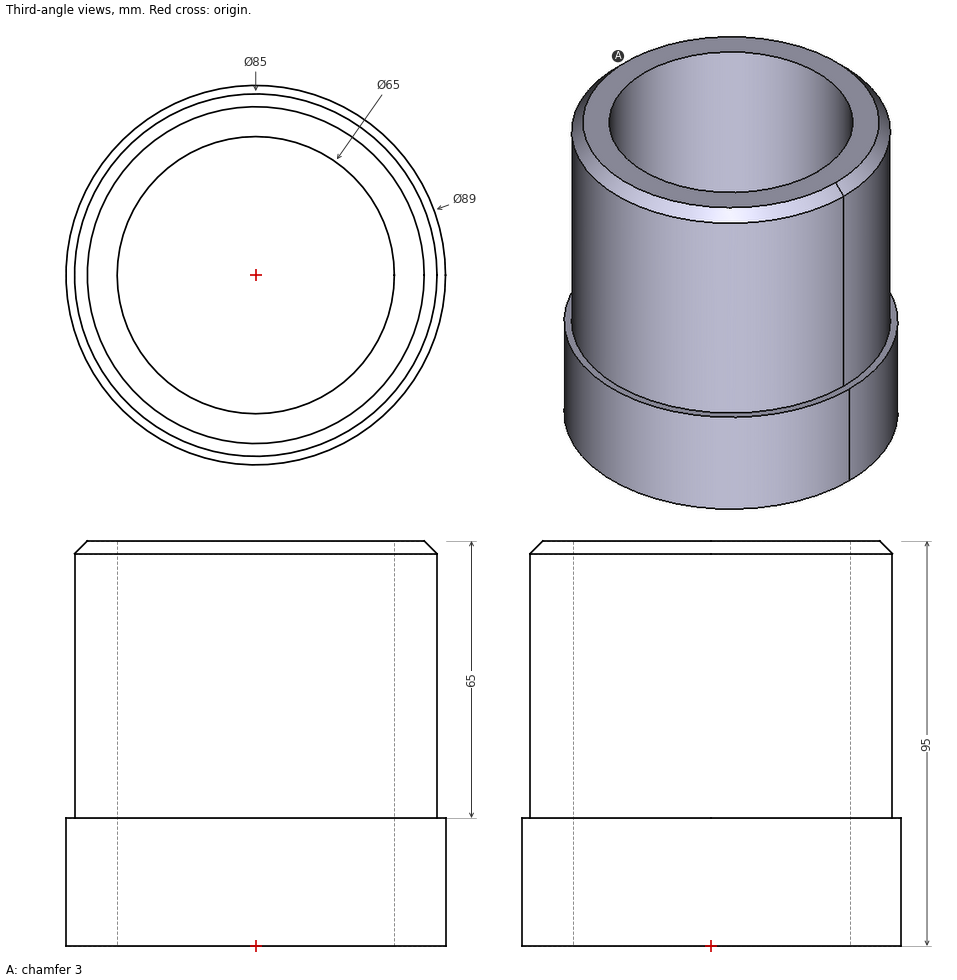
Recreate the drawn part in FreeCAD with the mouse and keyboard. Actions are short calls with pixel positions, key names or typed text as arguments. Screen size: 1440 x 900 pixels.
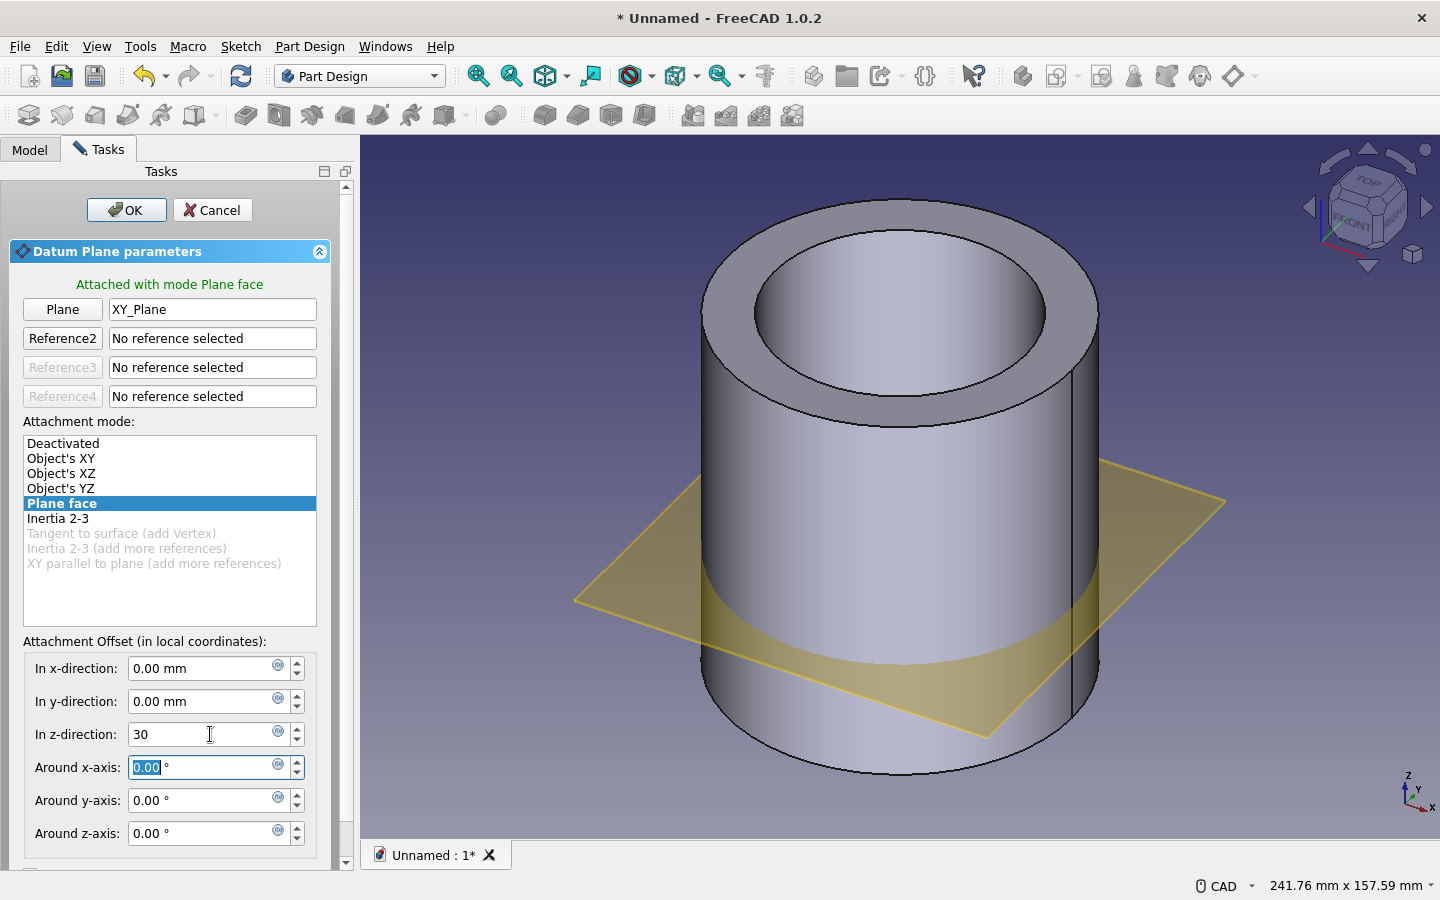
click(127, 210)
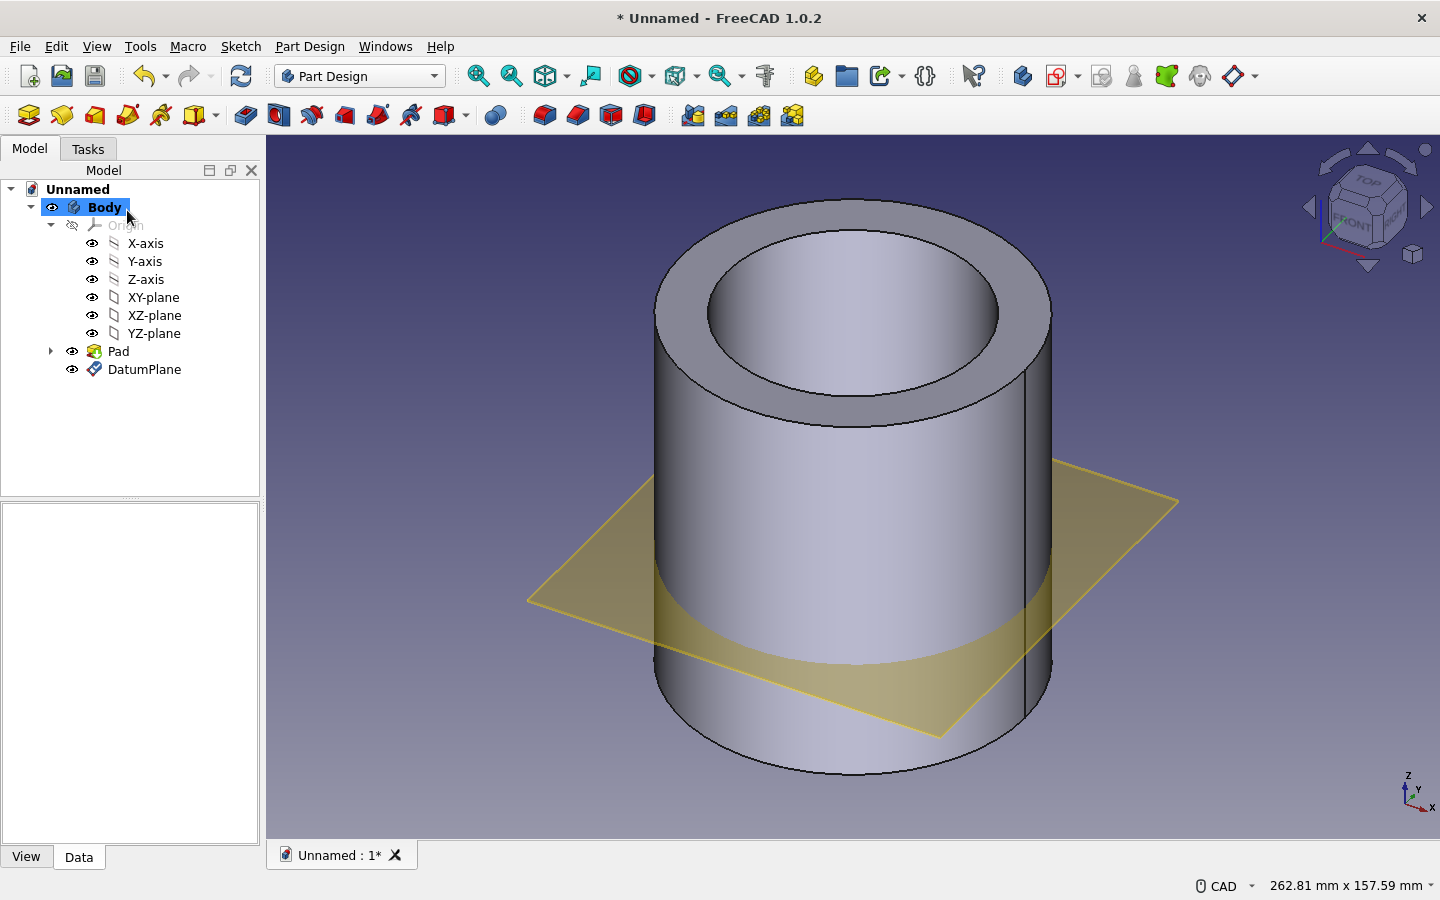
click(117, 369)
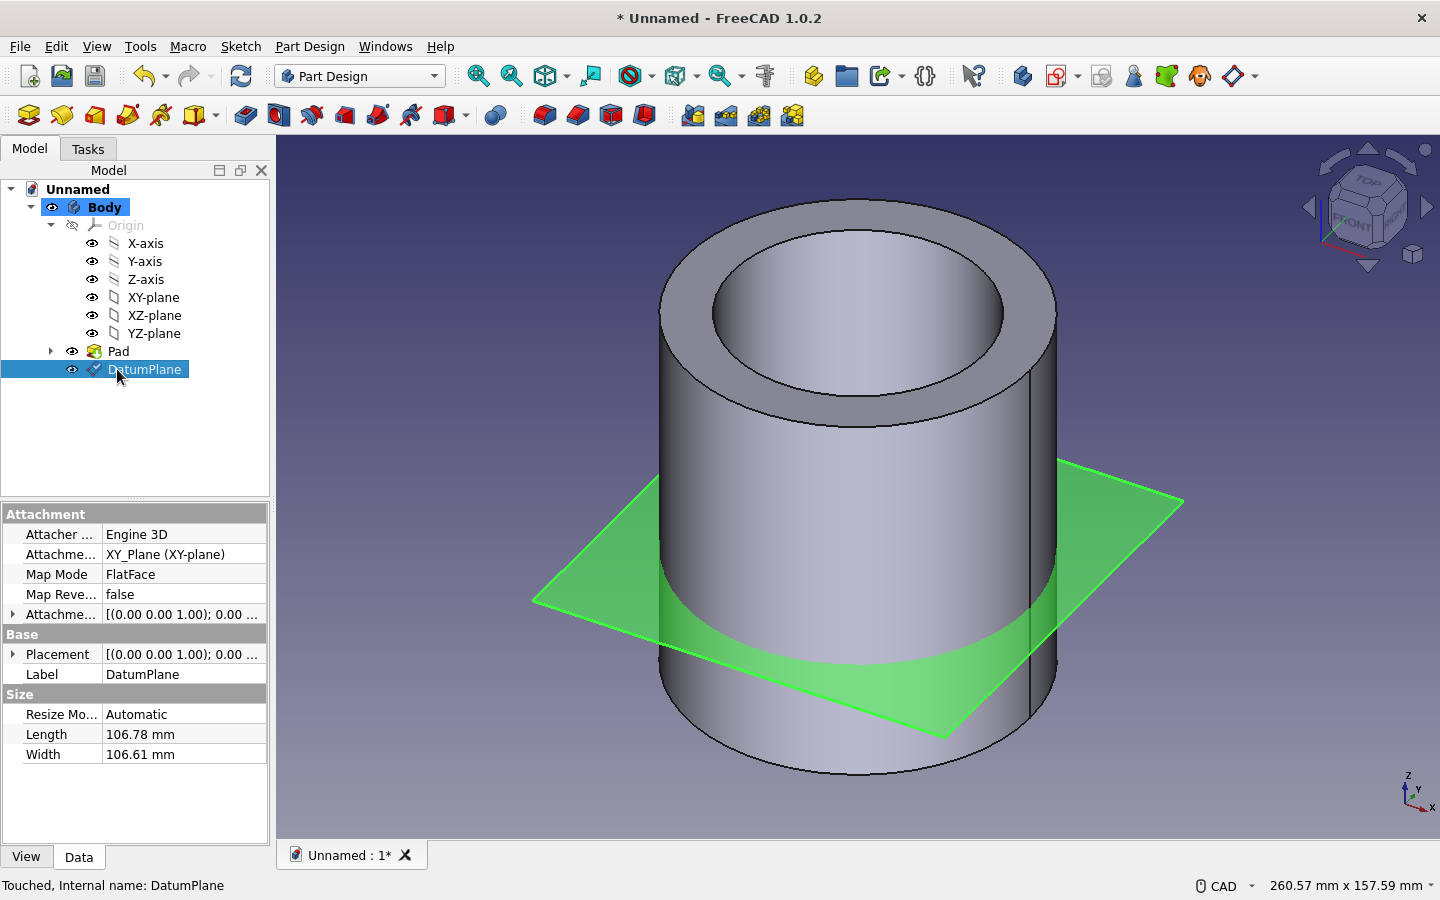
click(1056, 76)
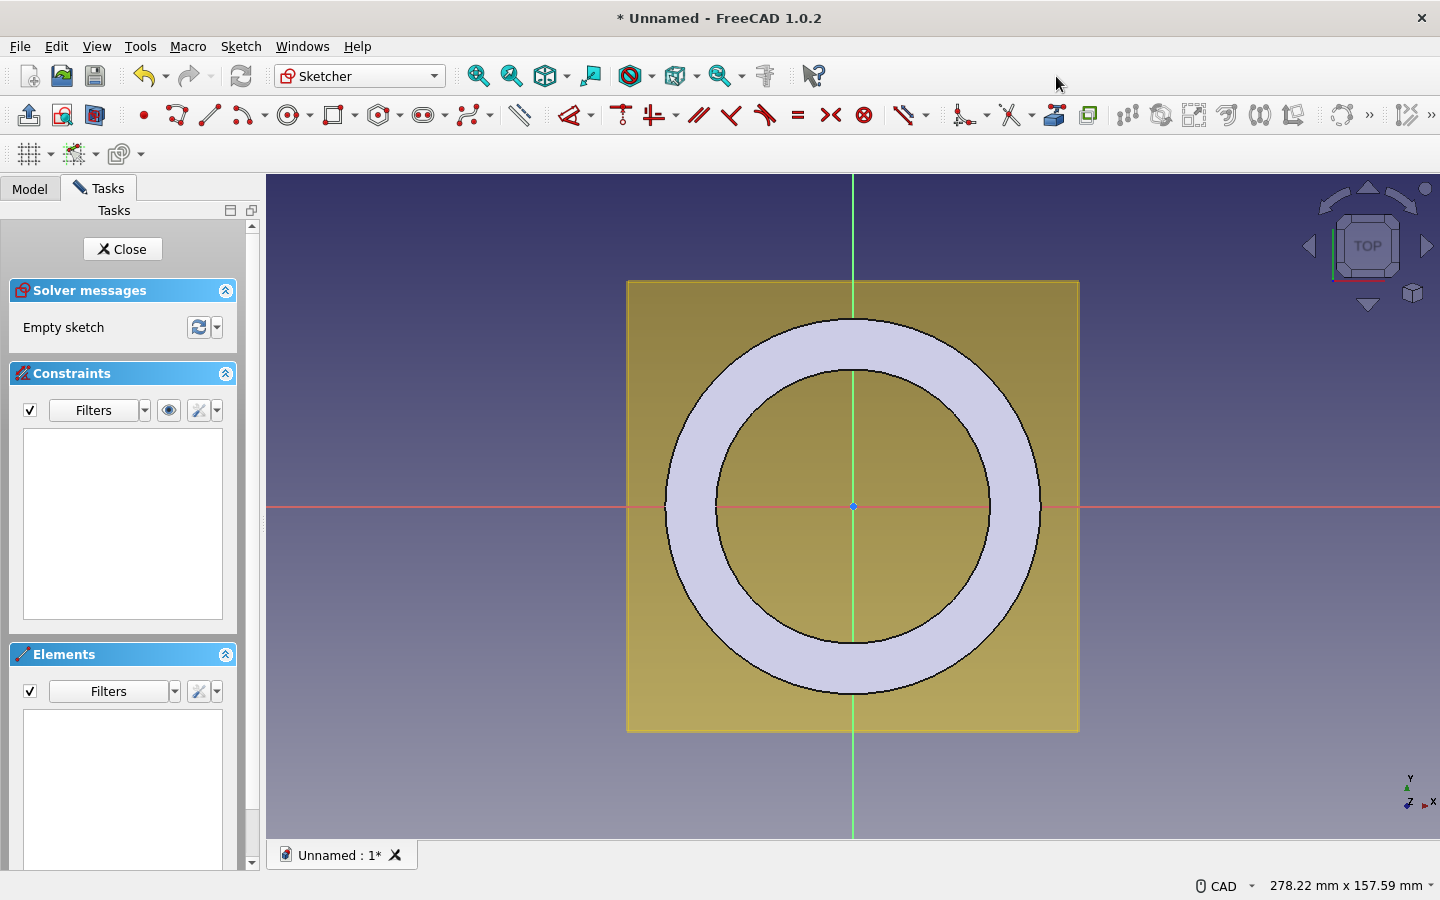
click(95, 116)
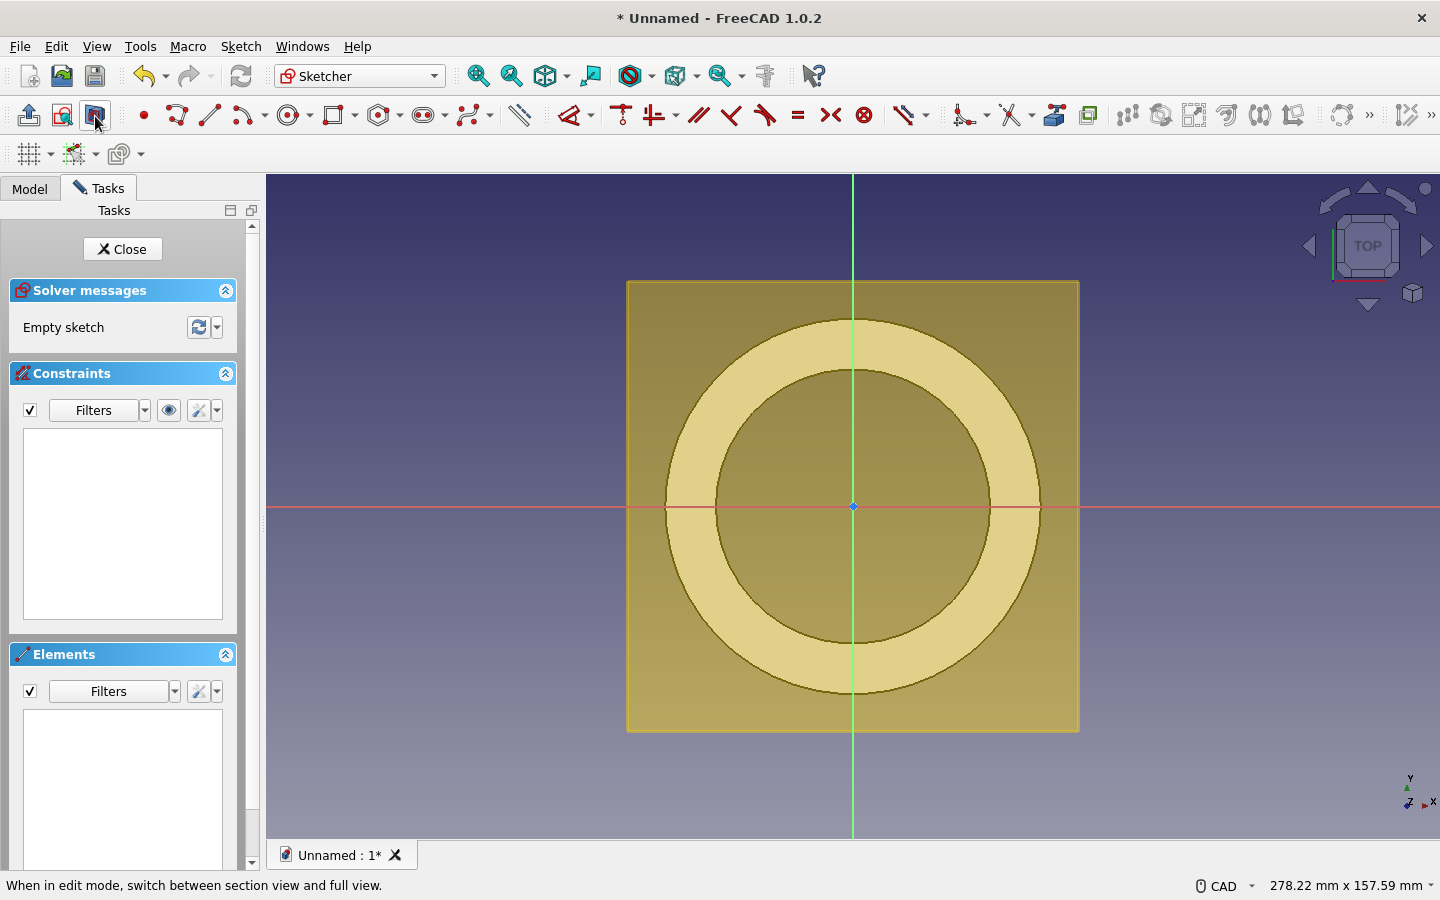
click(288, 116)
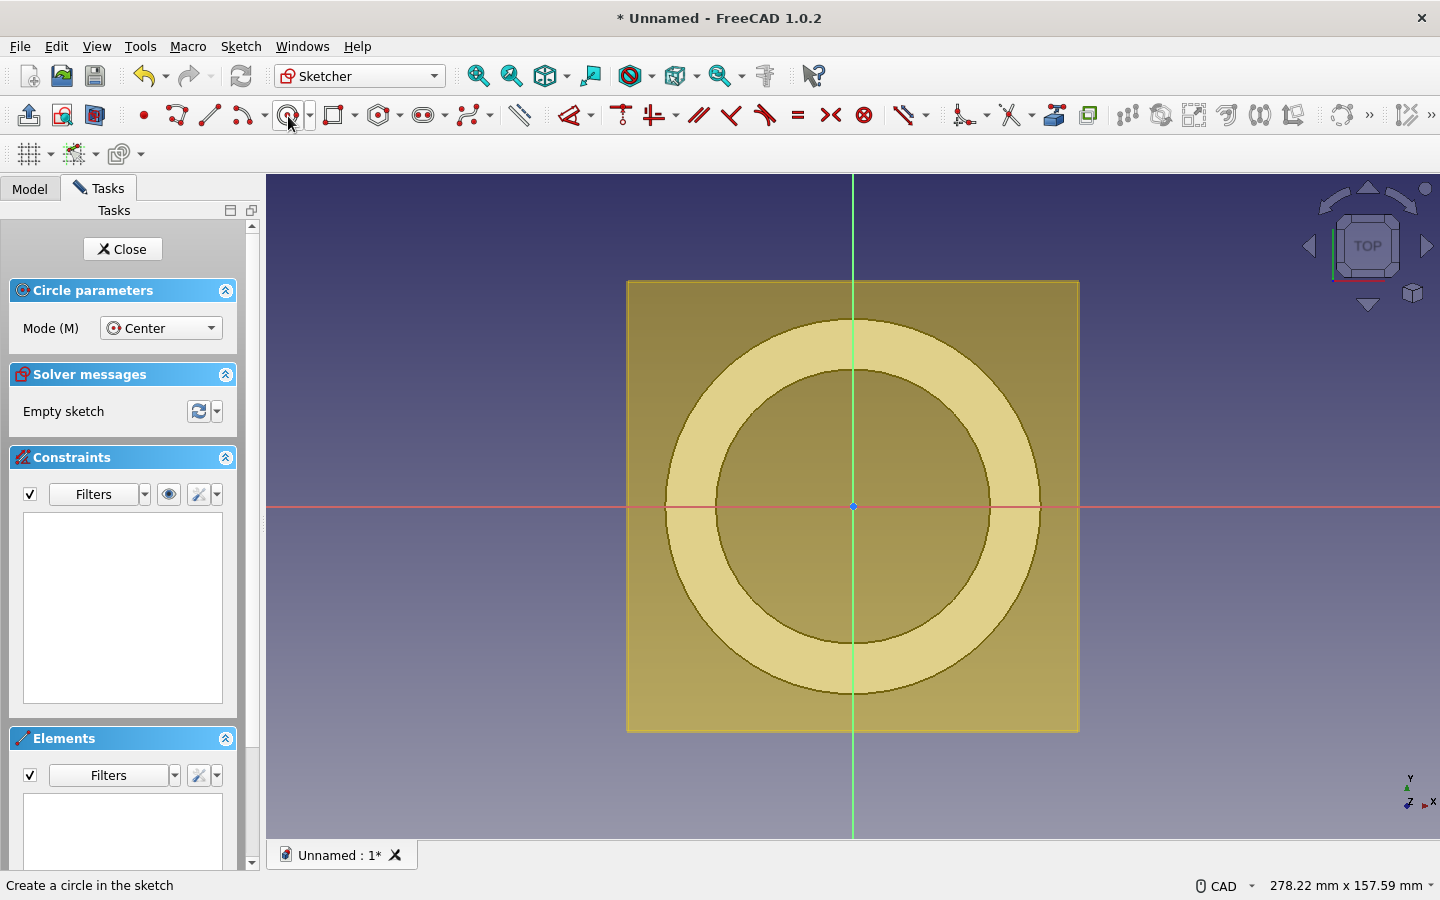
click(853, 506)
click(986, 374)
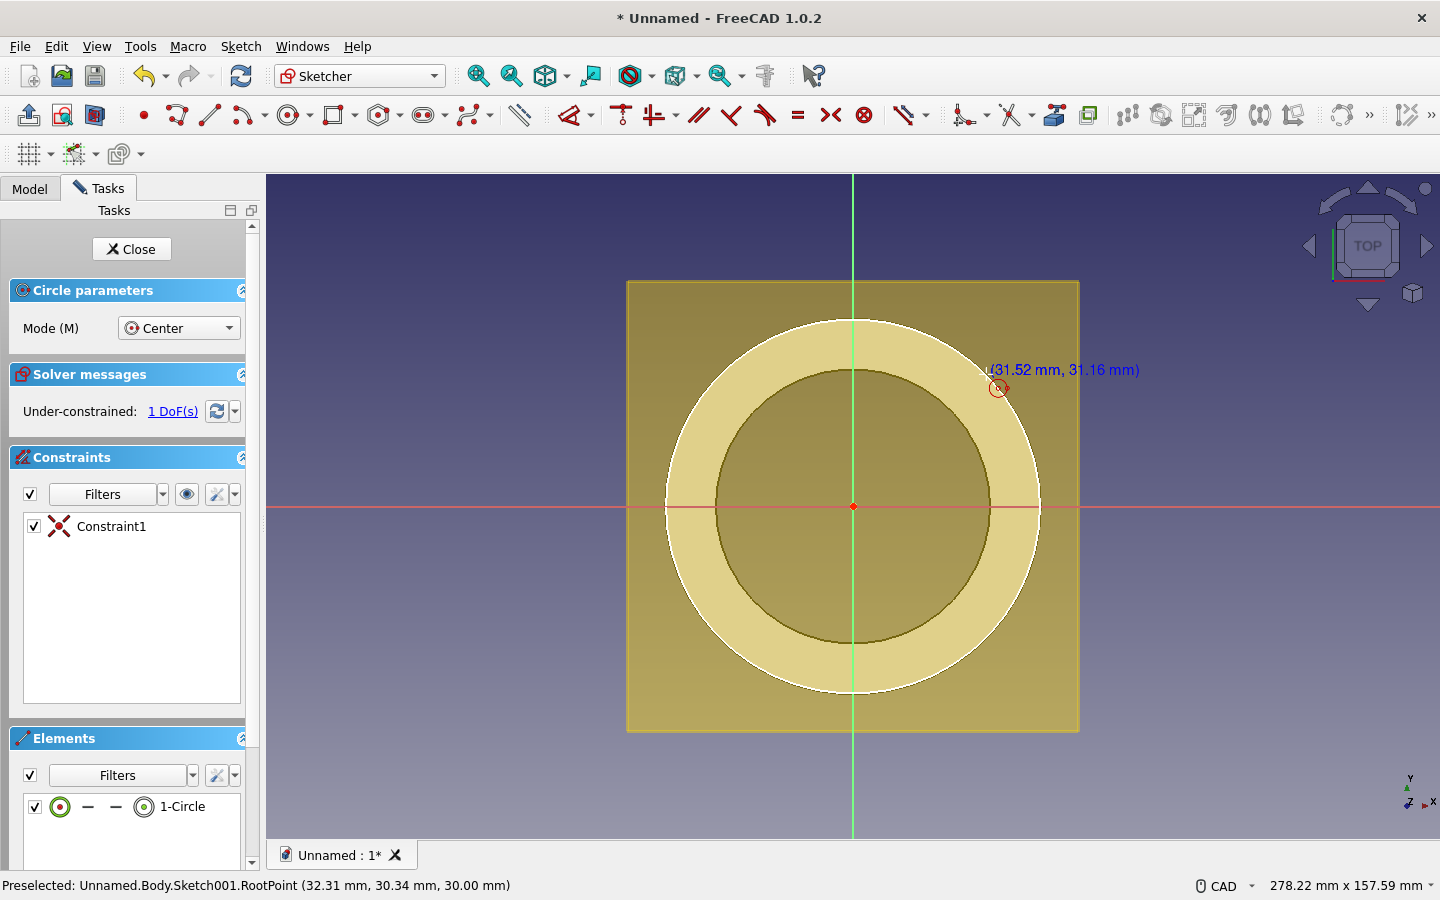
click(853, 506)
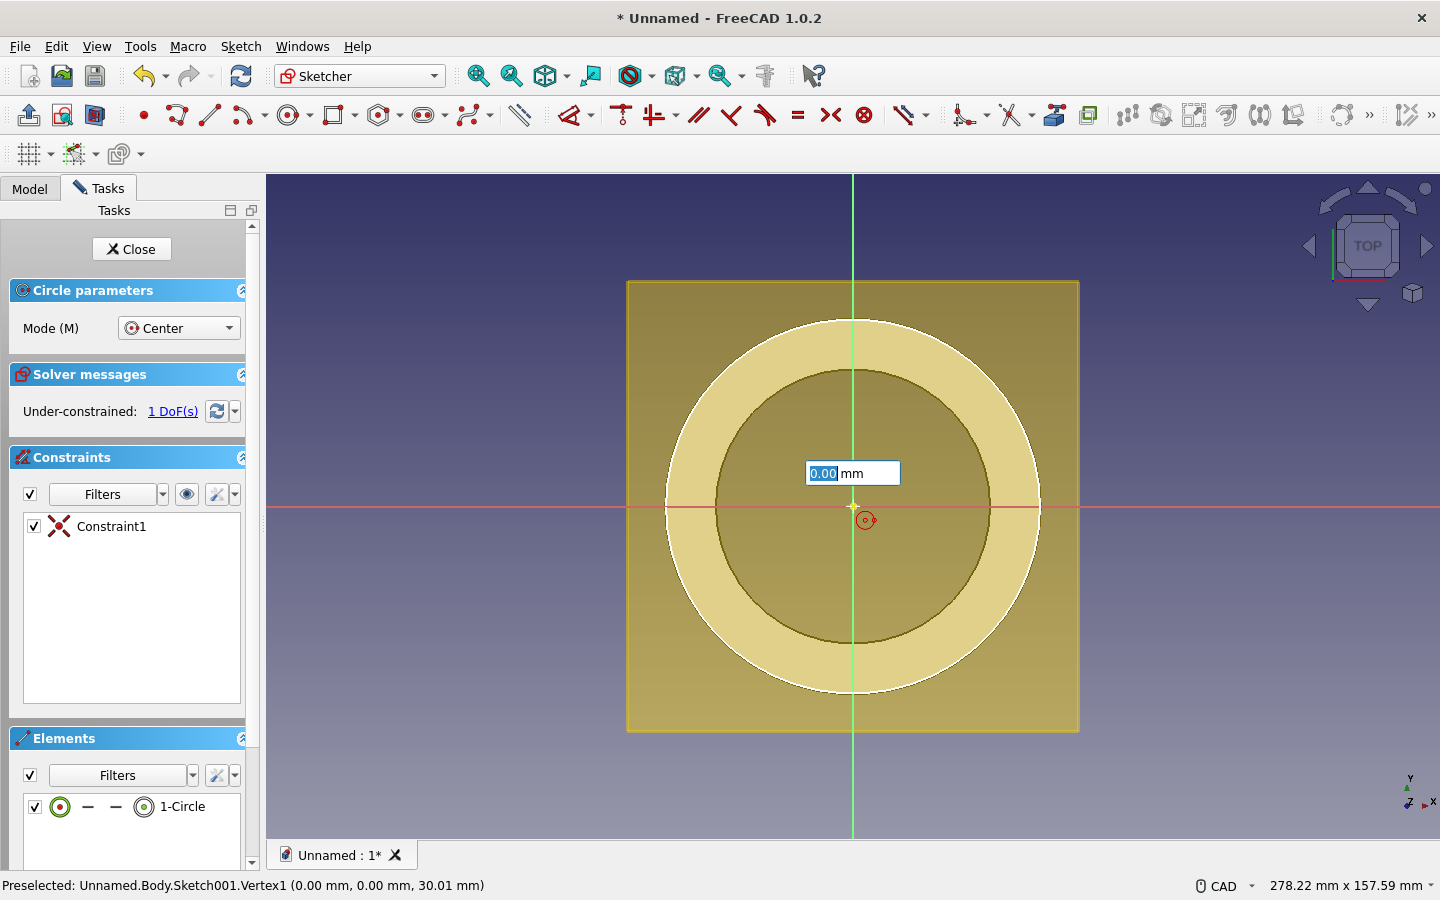
scroll(980, 380, up, 4)